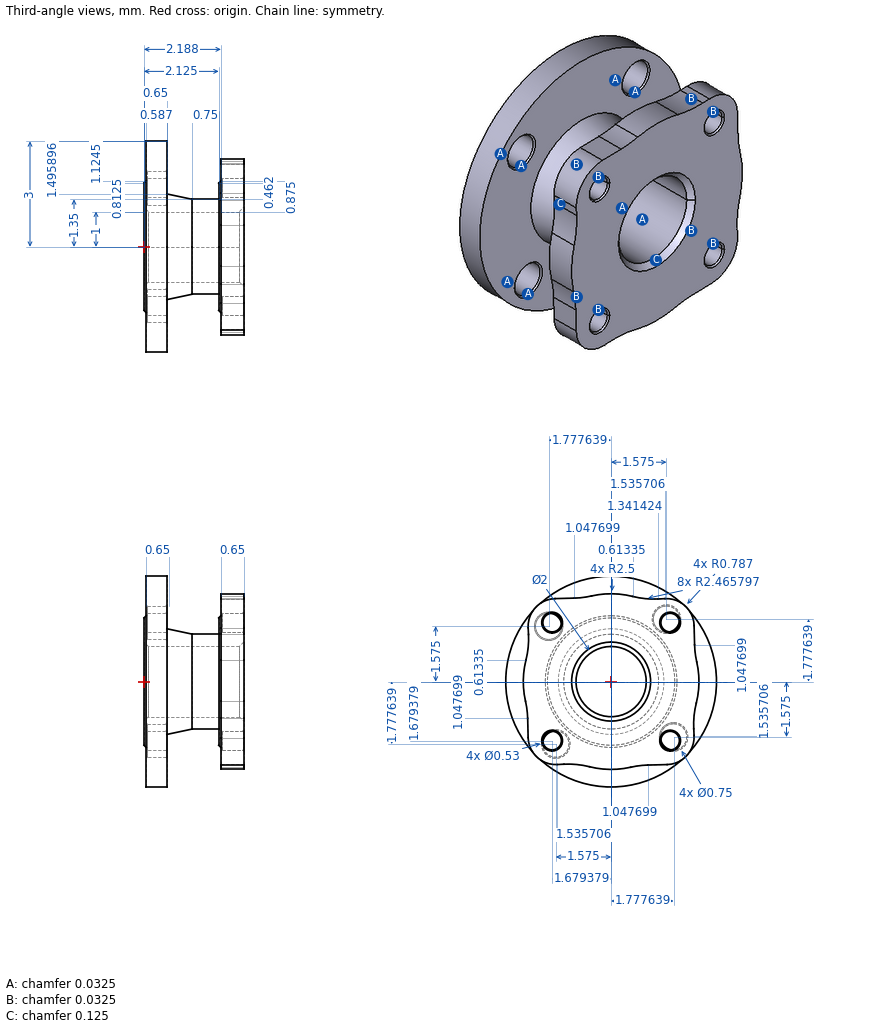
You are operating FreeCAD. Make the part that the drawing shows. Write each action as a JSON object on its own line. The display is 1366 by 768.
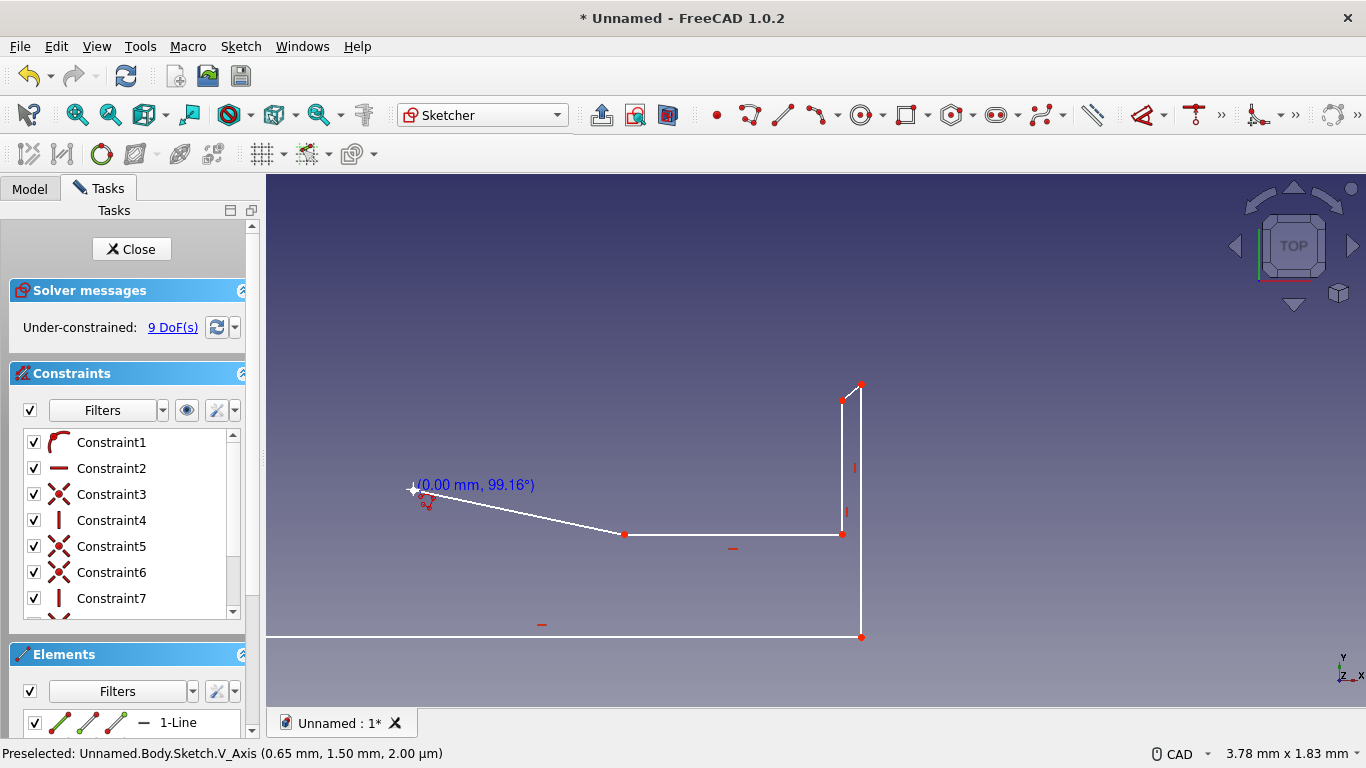
{"action": "scroll", "coordinate": [867, 411], "scroll_direction": "down", "scroll_amount": 5}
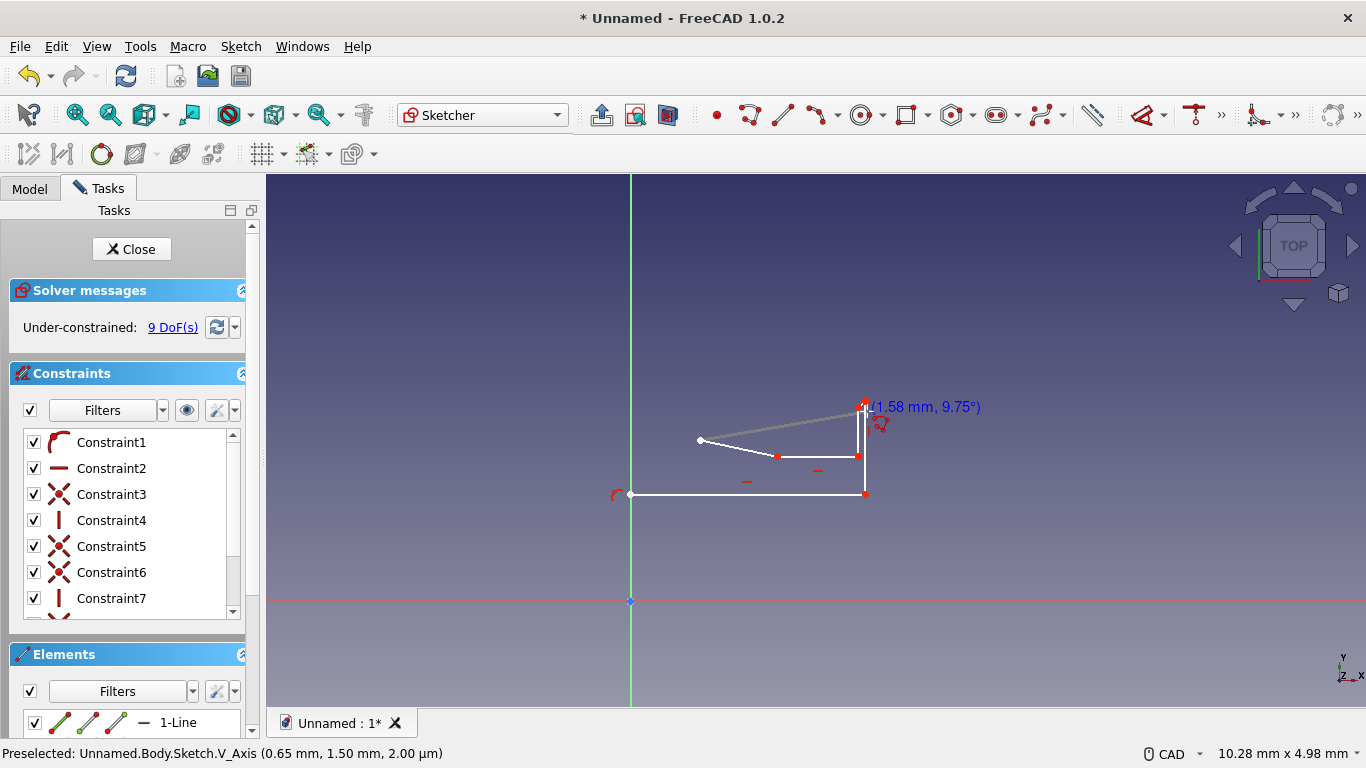
{"action": "left_click", "coordinate": [700, 280]}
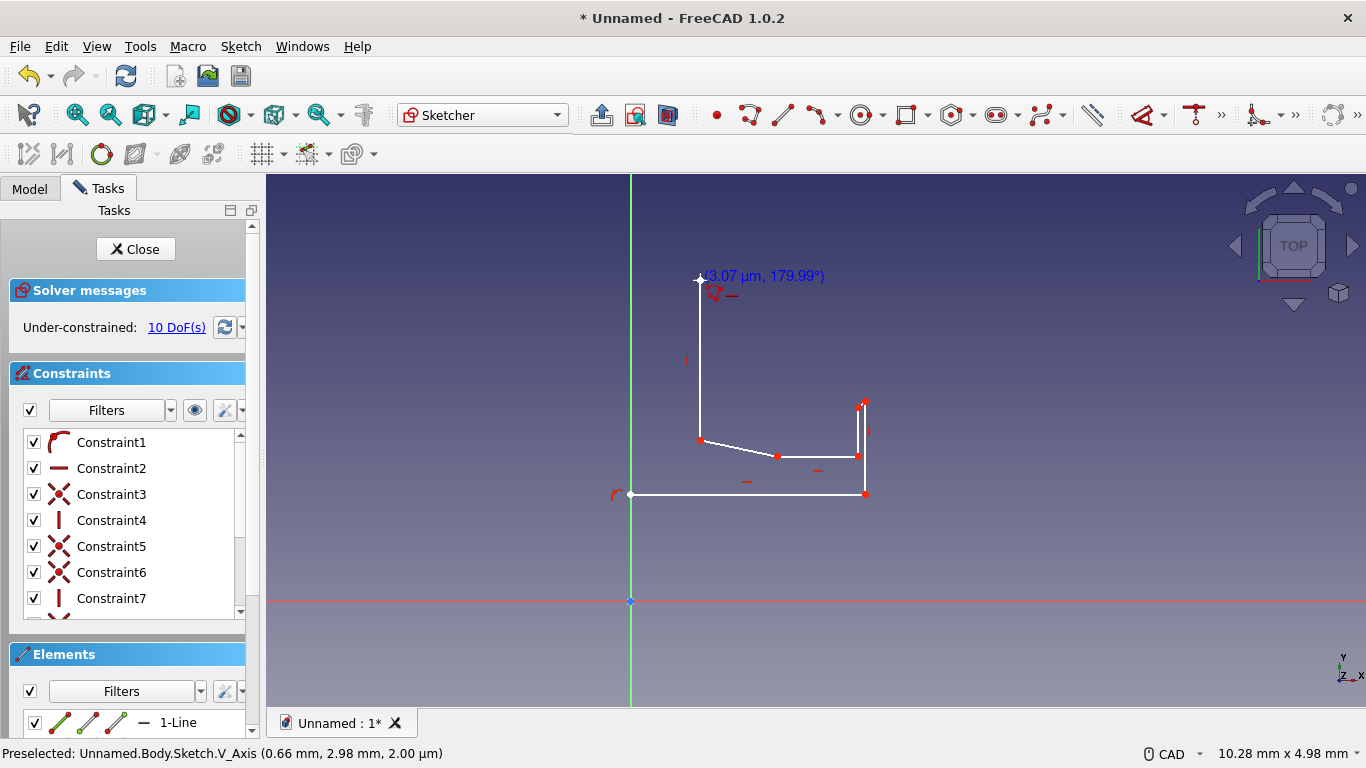
{"action": "scroll", "coordinate": [637, 280], "scroll_direction": "up", "scroll_amount": 5}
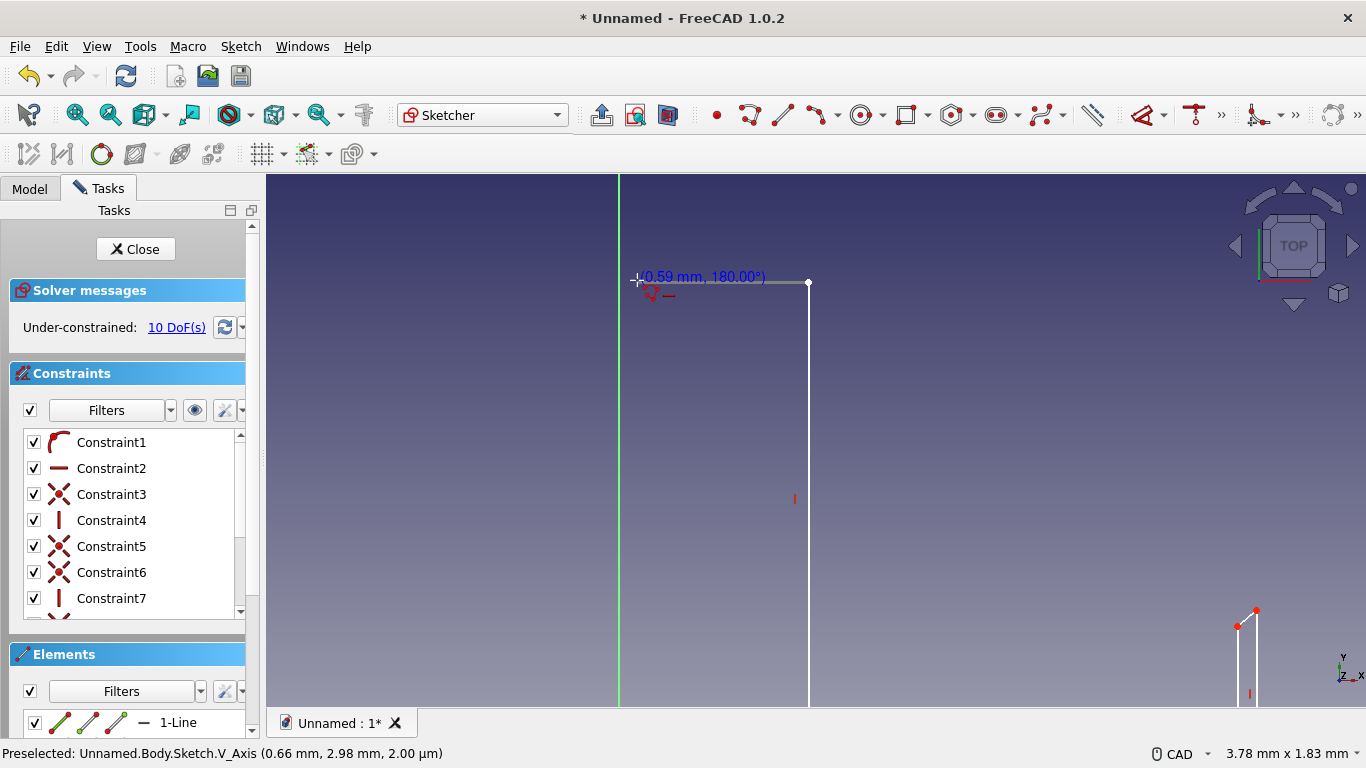
{"action": "left_click", "coordinate": [637, 280]}
{"action": "left_click", "coordinate": [637, 607]}
{"action": "left_click", "coordinate": [628, 625]}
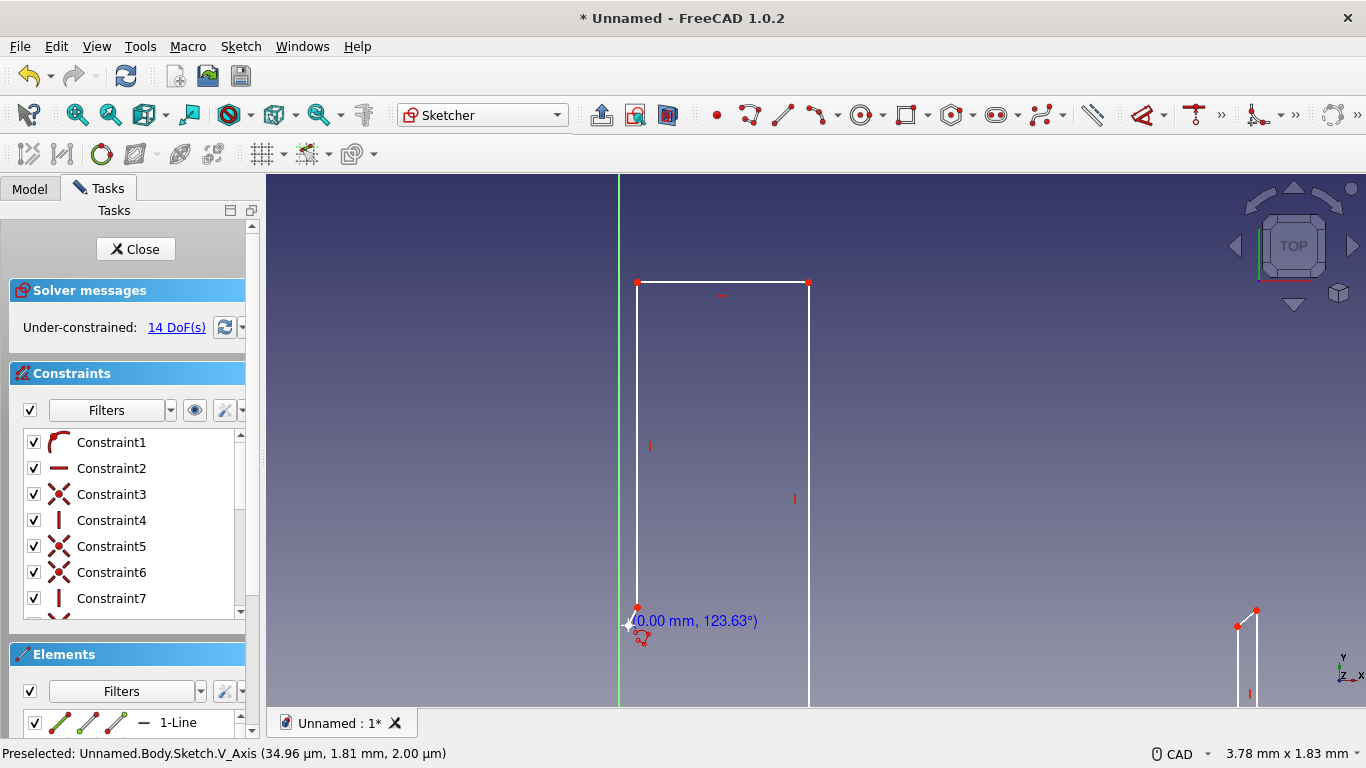
{"action": "scroll", "coordinate": [637, 280], "scroll_direction": "down", "scroll_amount": 5}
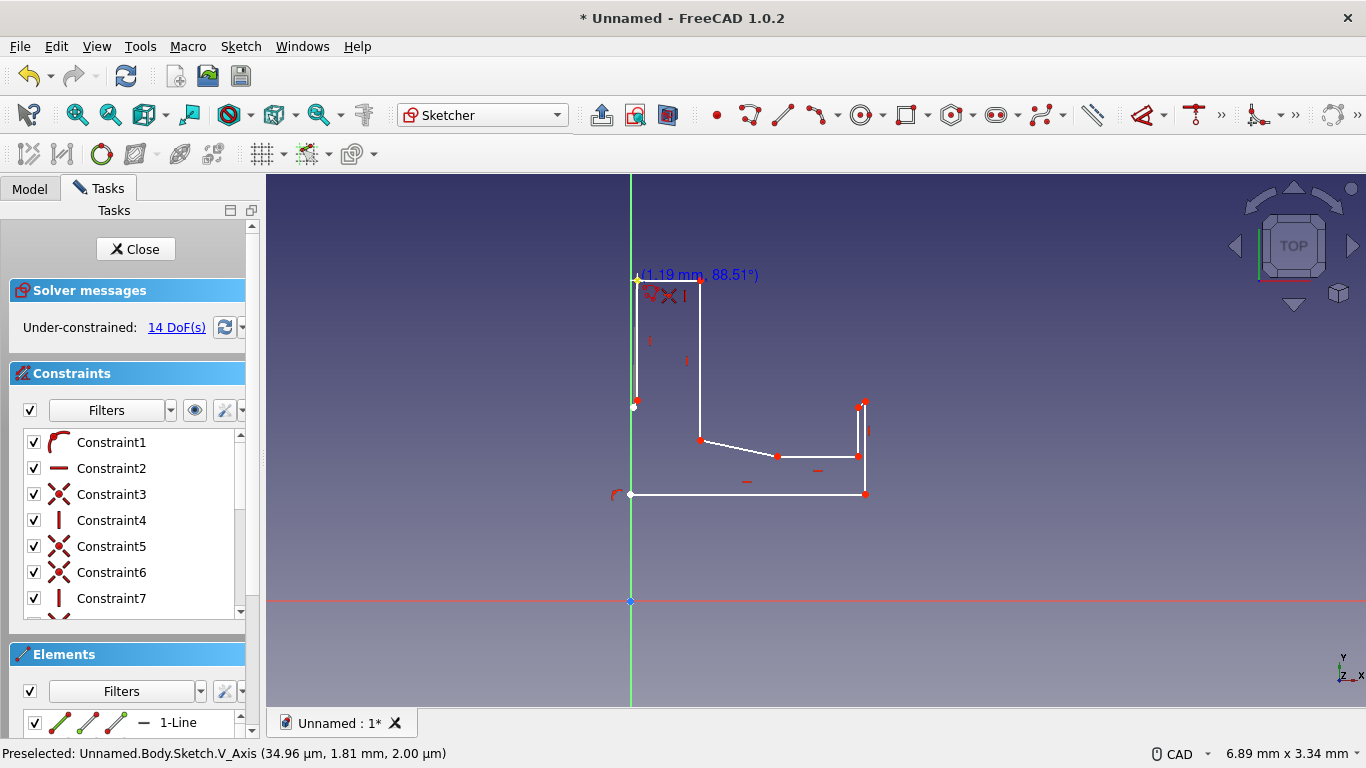
{"action": "left_click", "coordinate": [631, 495]}
{"action": "key", "text": "Escape"}
{"action": "key", "text": "Escape"}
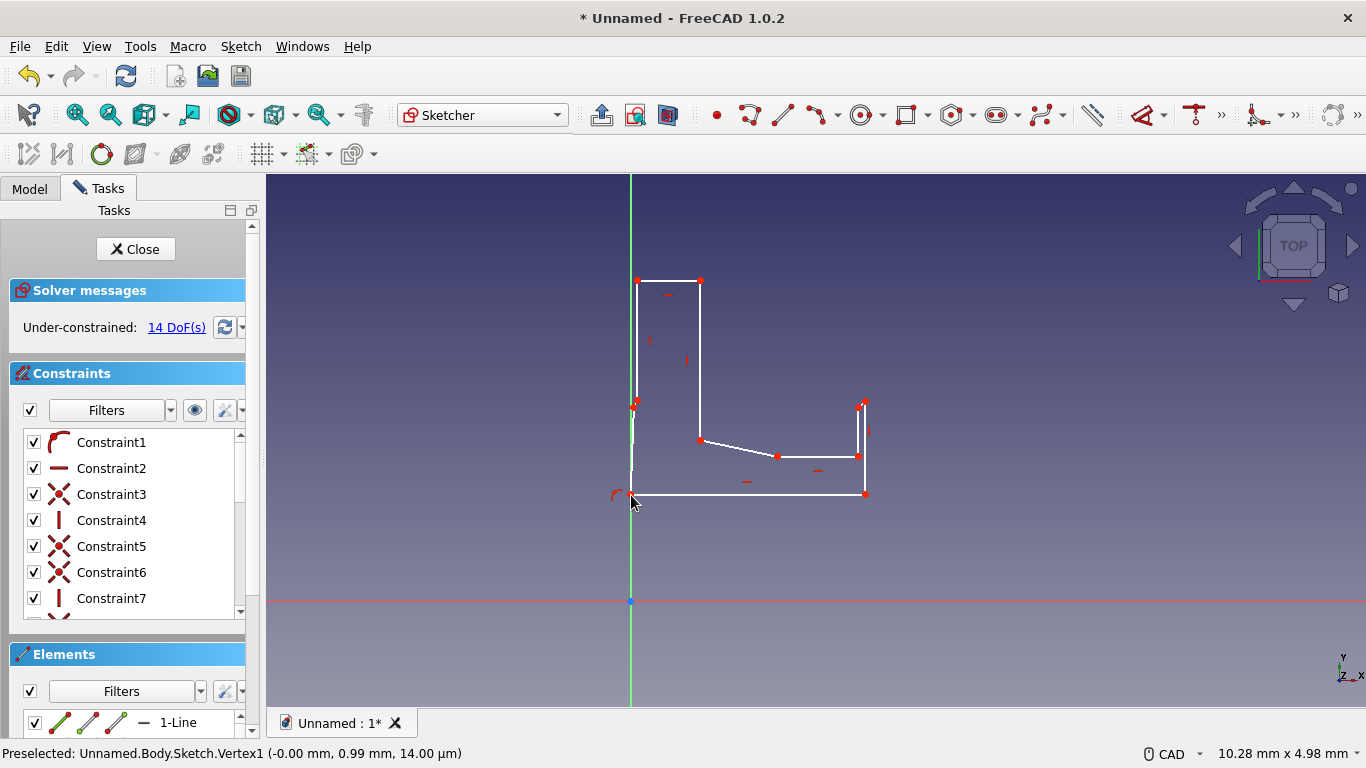
{"action": "left_click", "coordinate": [633, 434]}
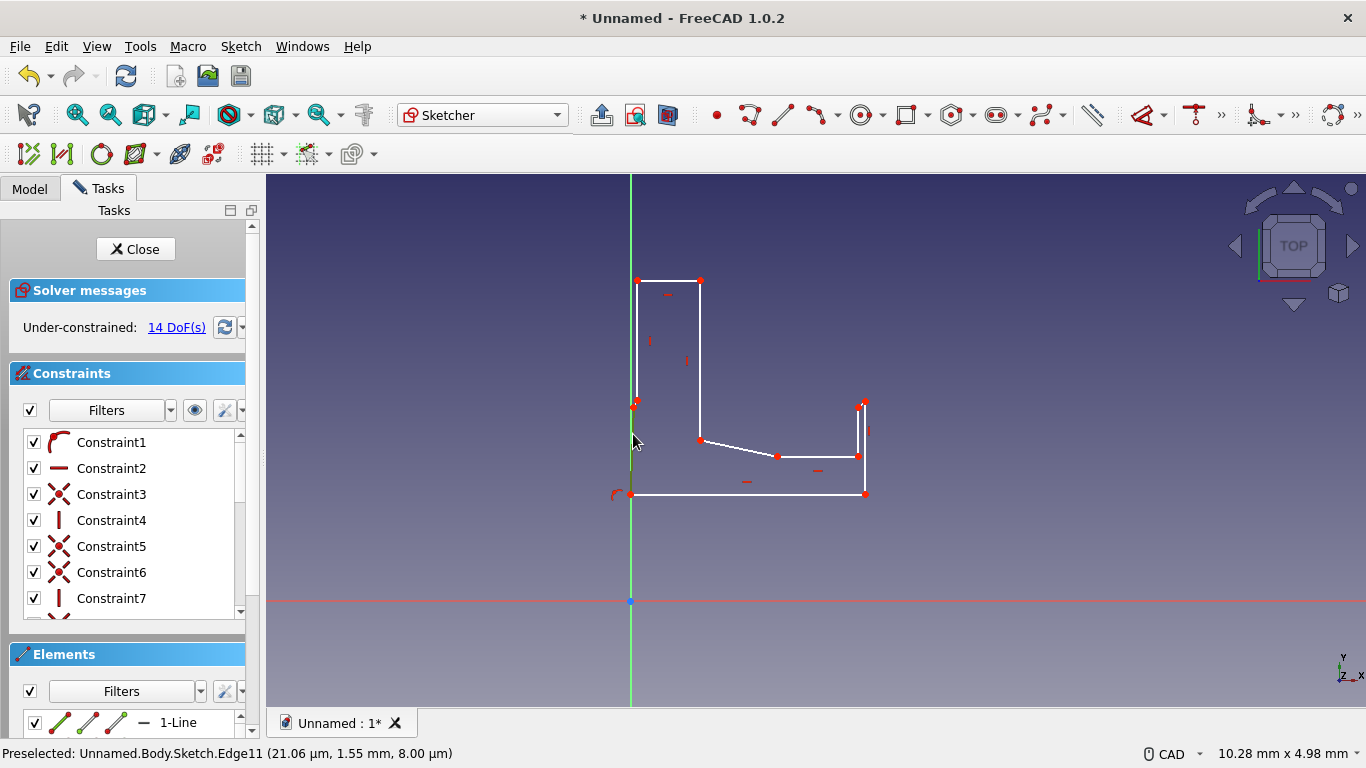
{"action": "key", "text": "v"}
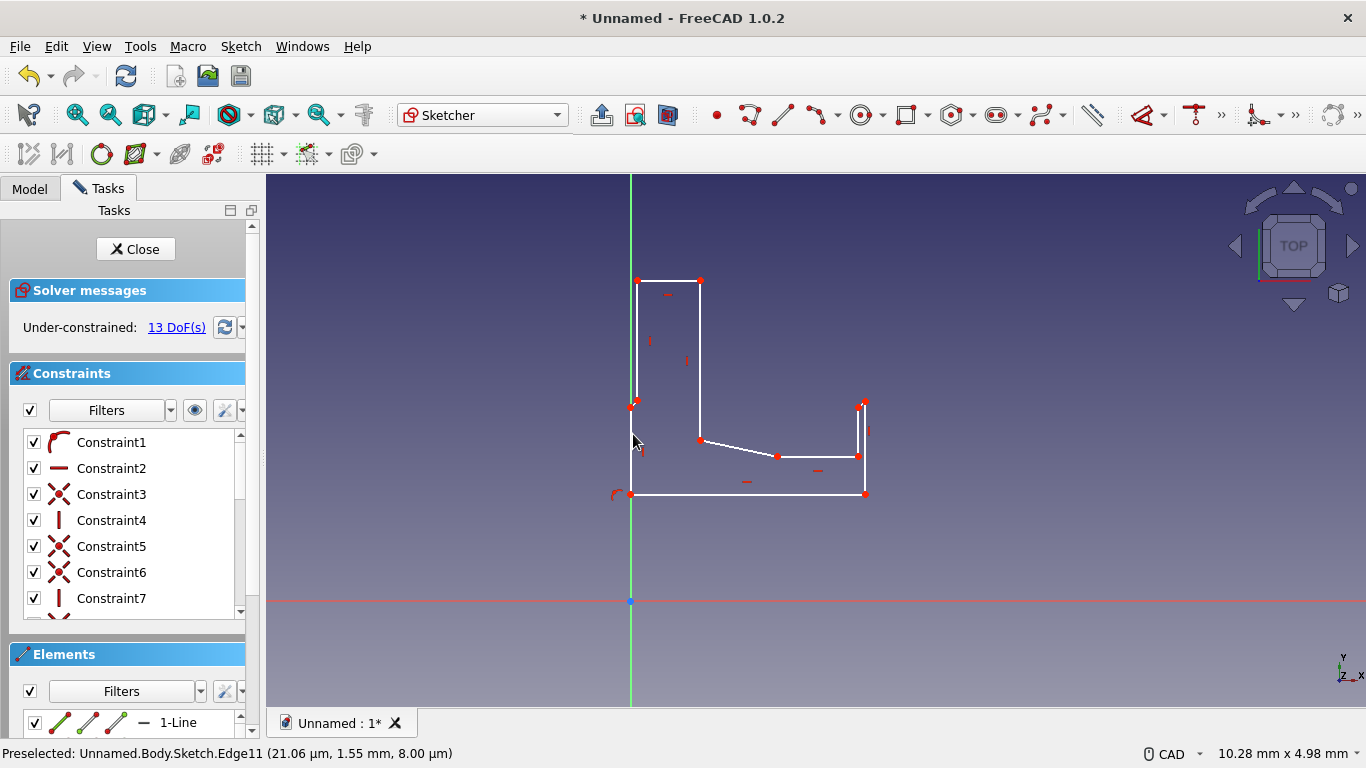
{"action": "left_click", "coordinate": [1142, 116]}